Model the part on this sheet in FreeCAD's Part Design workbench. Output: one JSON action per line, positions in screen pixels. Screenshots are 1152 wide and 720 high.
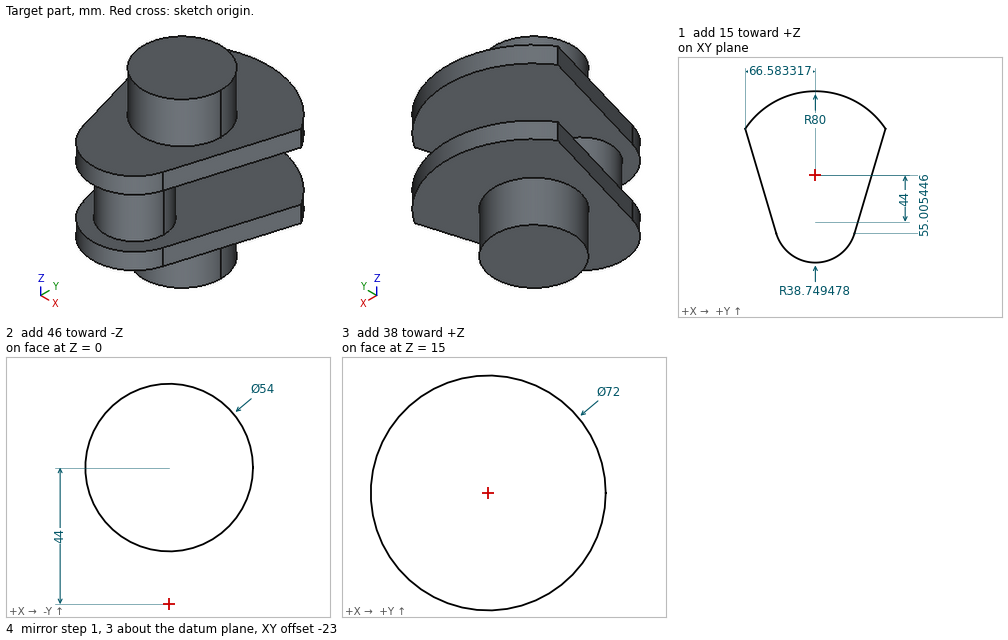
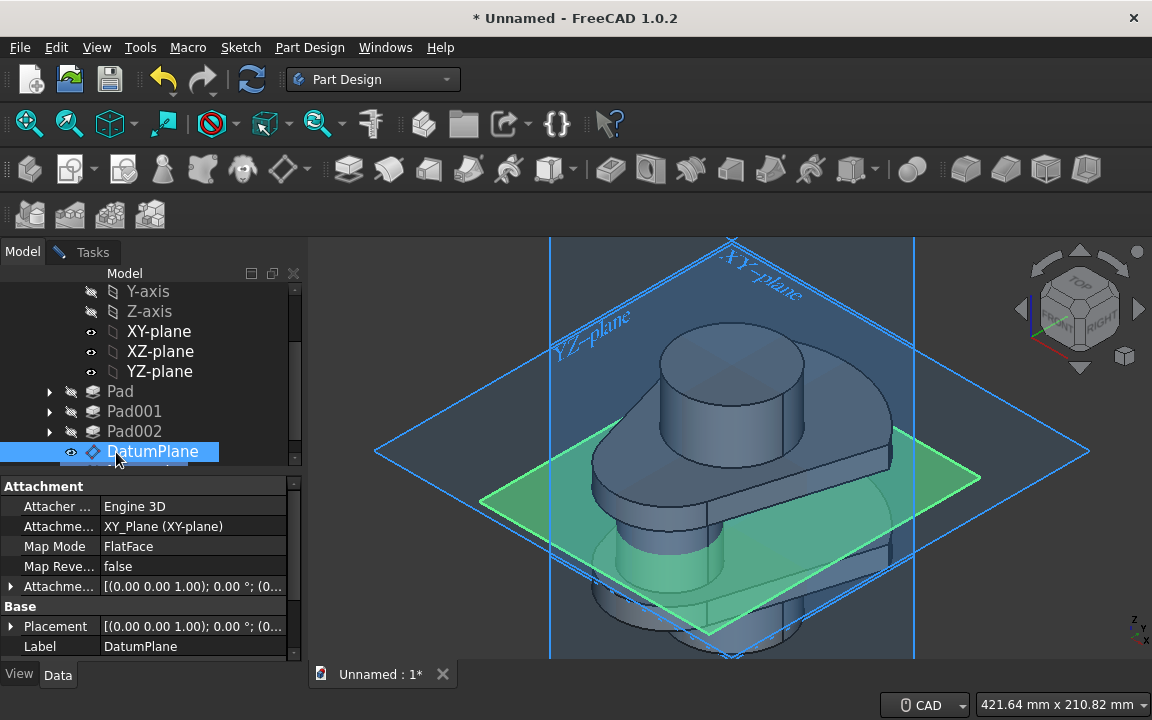
{"action": "left_click", "coordinate": [84, 251]}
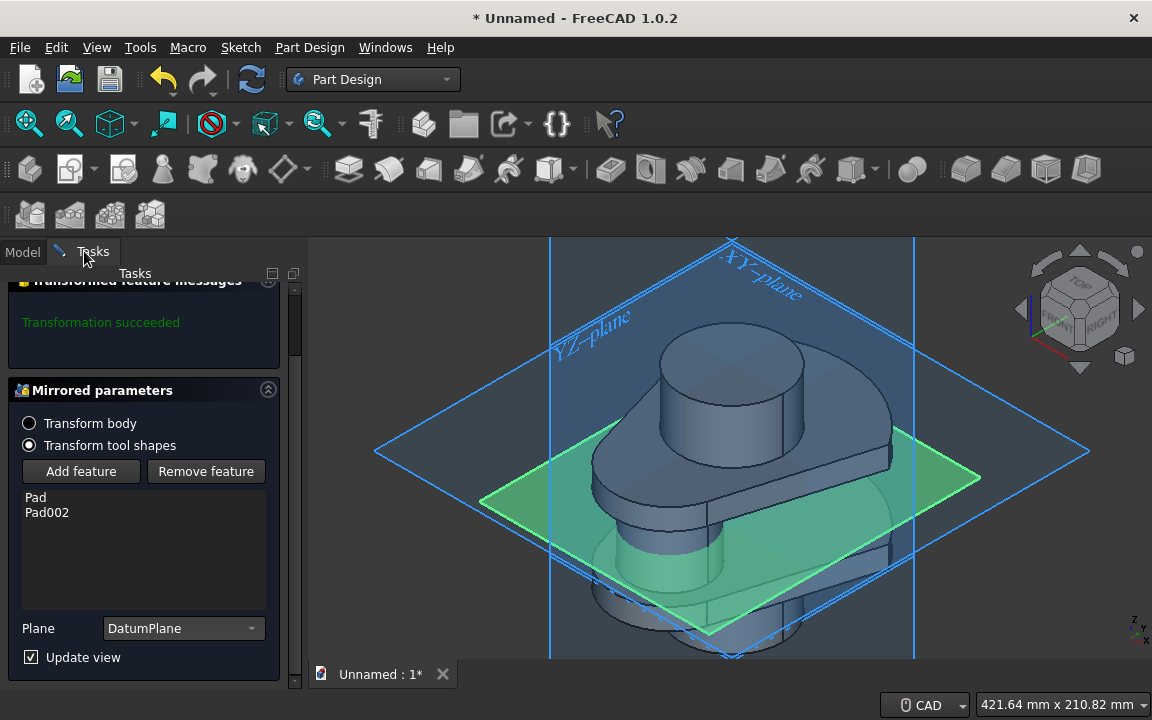
{"action": "scroll", "coordinate": [295, 486], "scroll_direction": "up", "scroll_amount": 2}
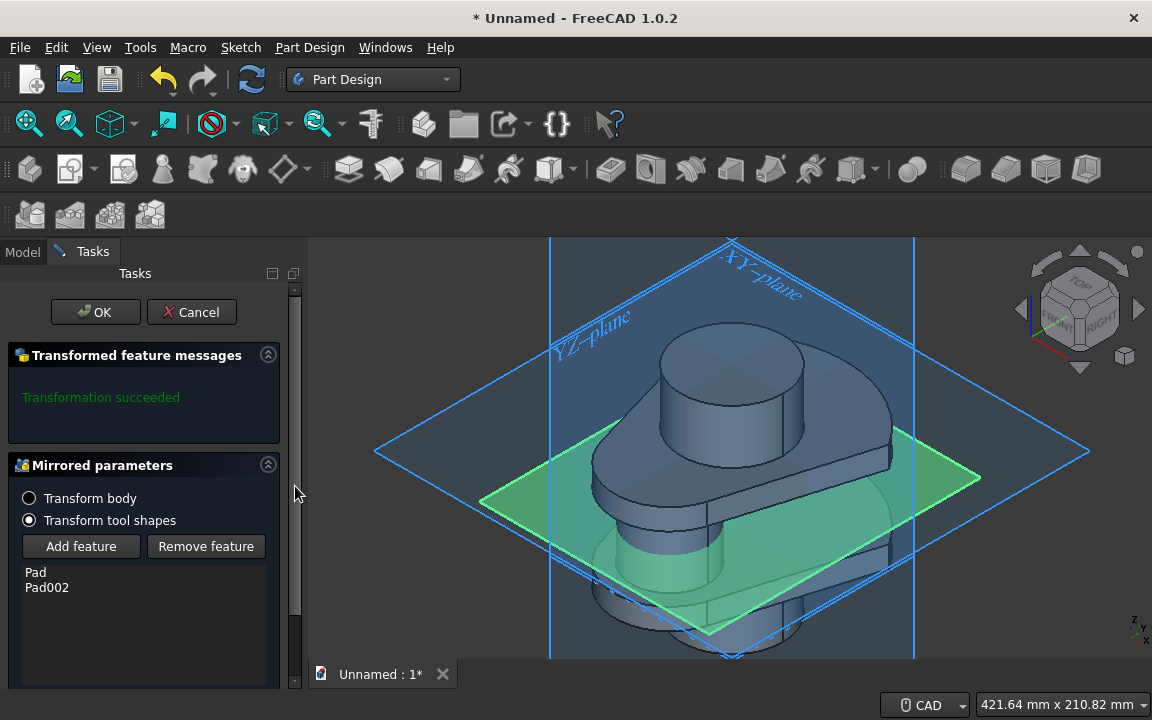
{"action": "left_click", "coordinate": [96, 312]}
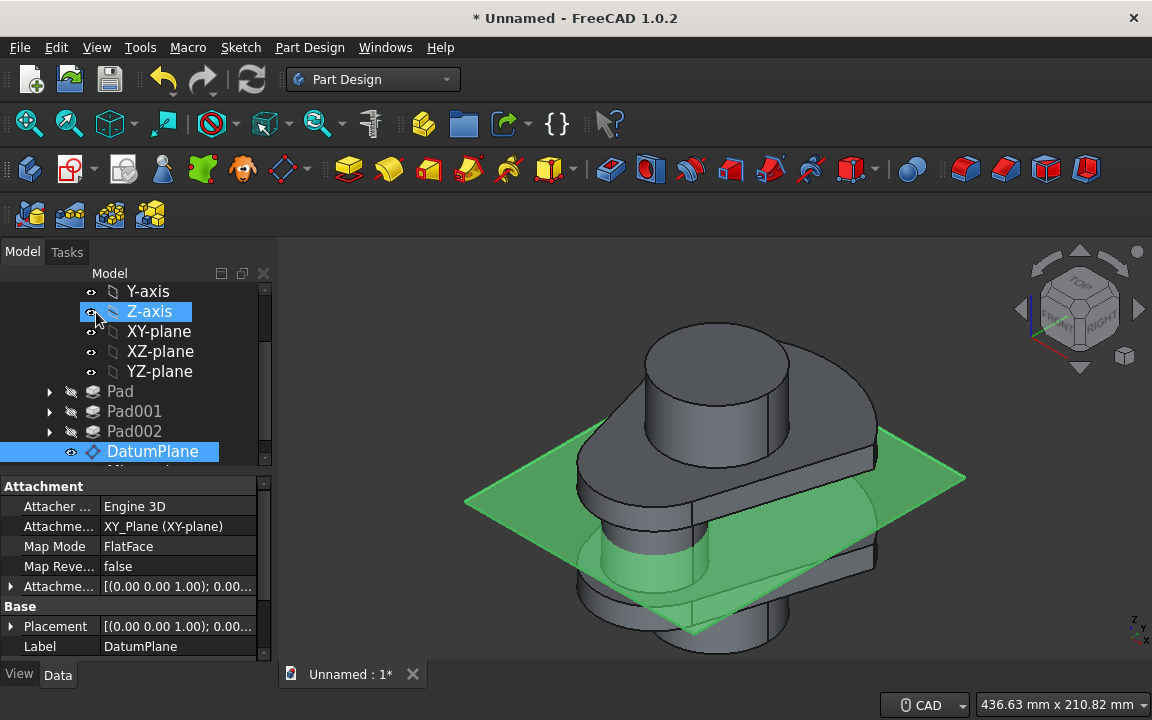
{"action": "left_click", "coordinate": [116, 452]}
{"action": "key", "text": "space"}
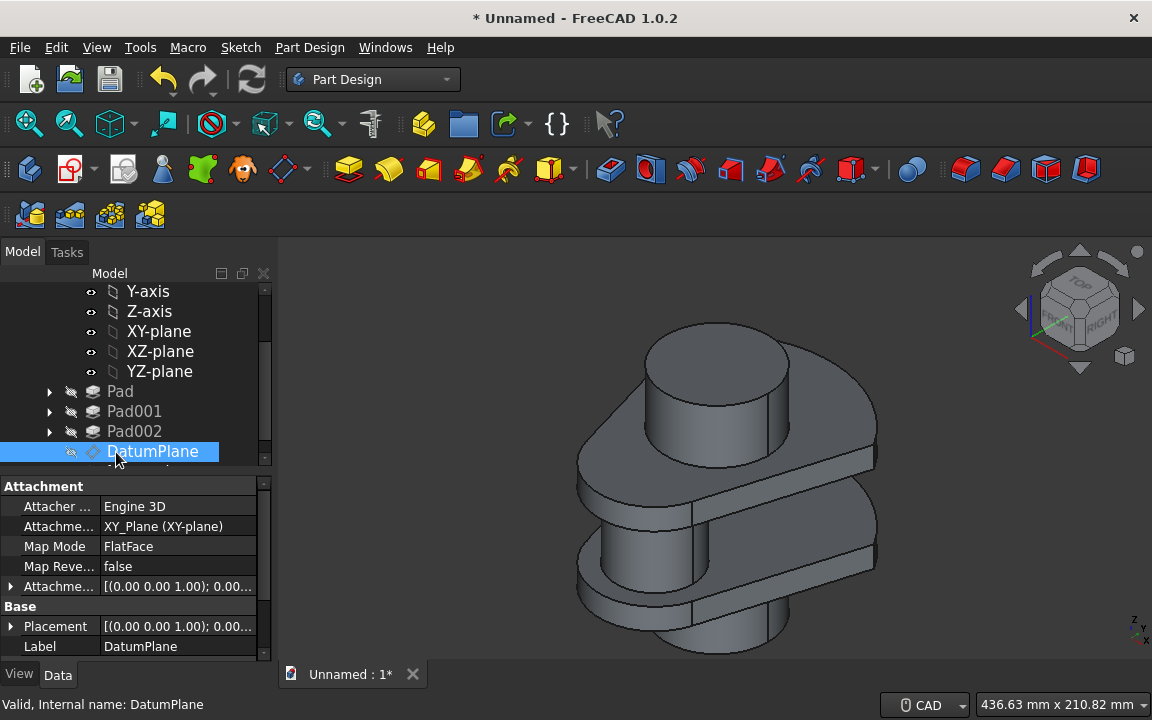
{"action": "left_click", "coordinate": [30, 124]}